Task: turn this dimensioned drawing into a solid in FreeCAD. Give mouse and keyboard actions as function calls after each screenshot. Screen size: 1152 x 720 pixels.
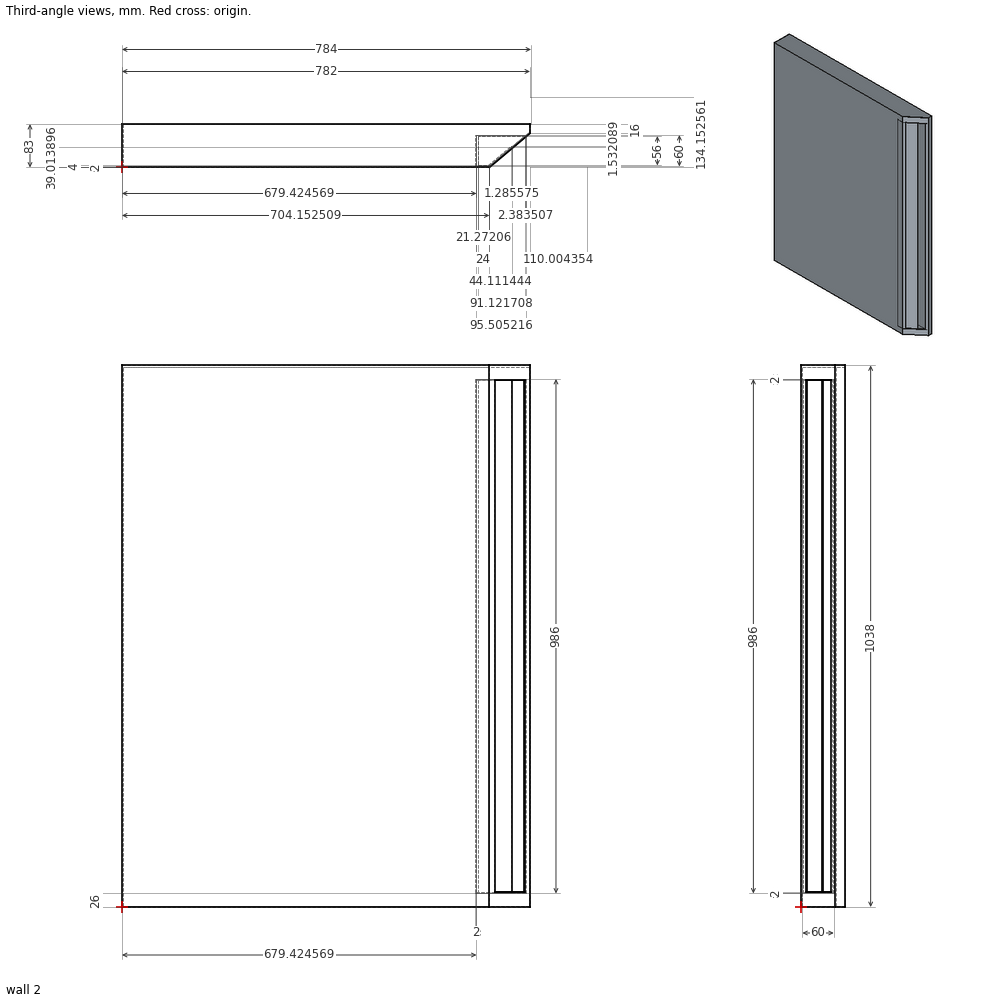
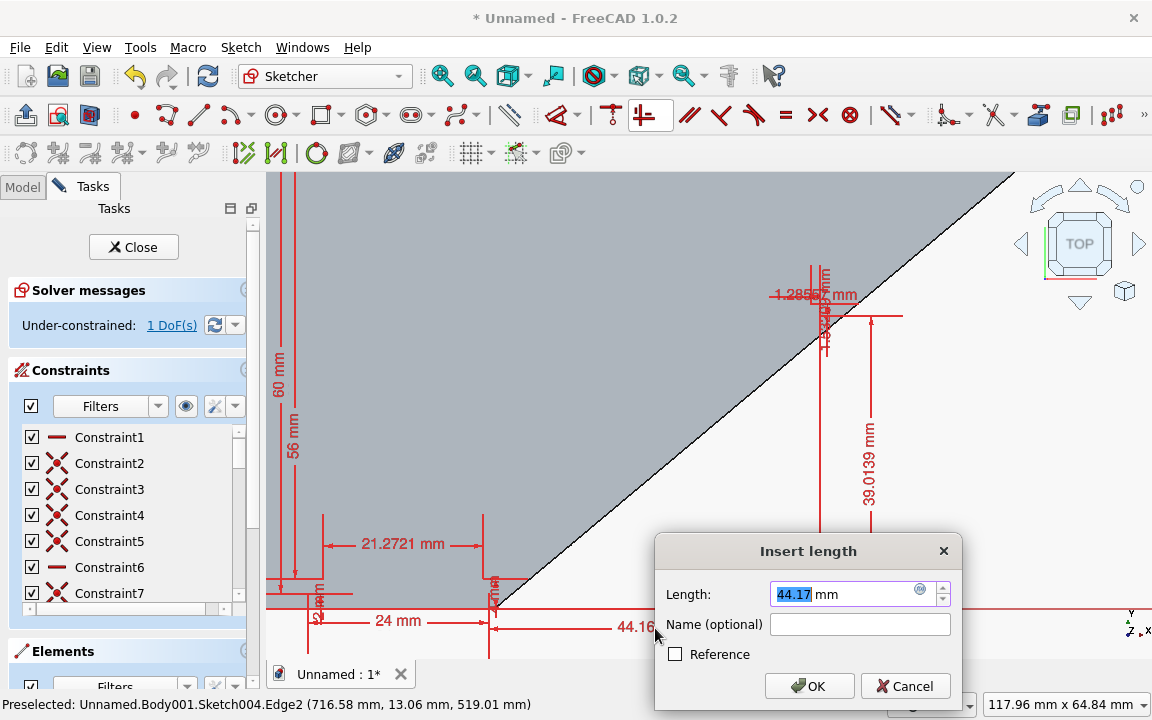
text(44.111444)
key(Return)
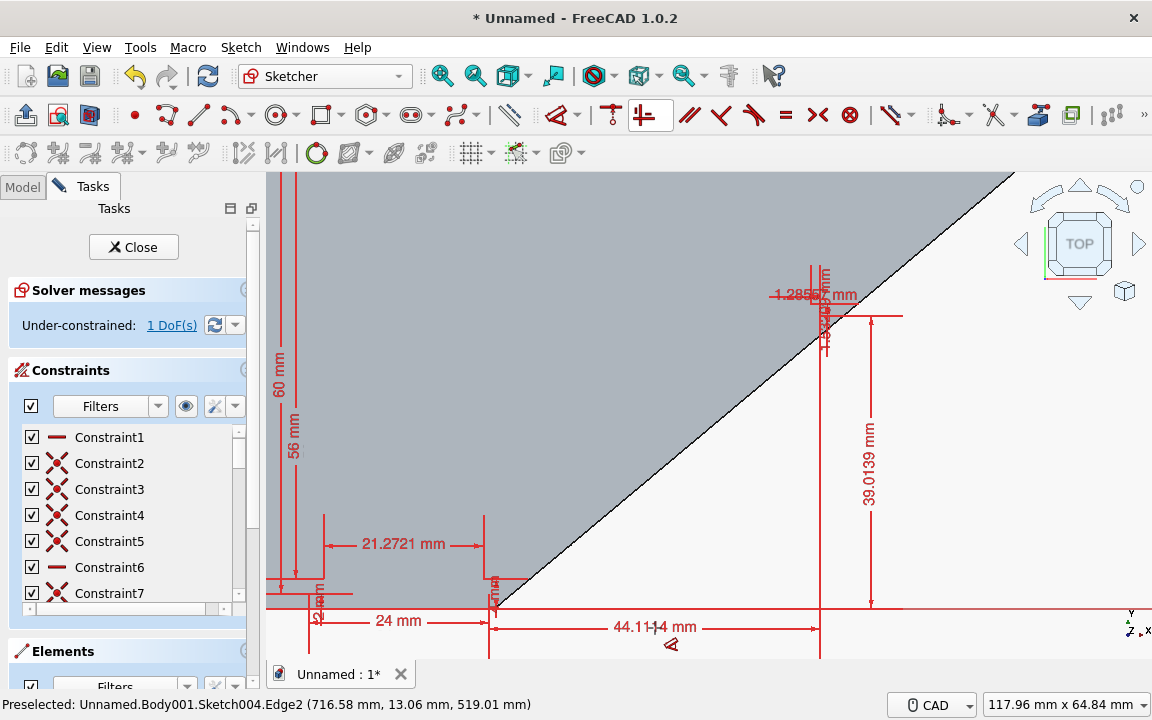
click(309, 594)
click(301, 560)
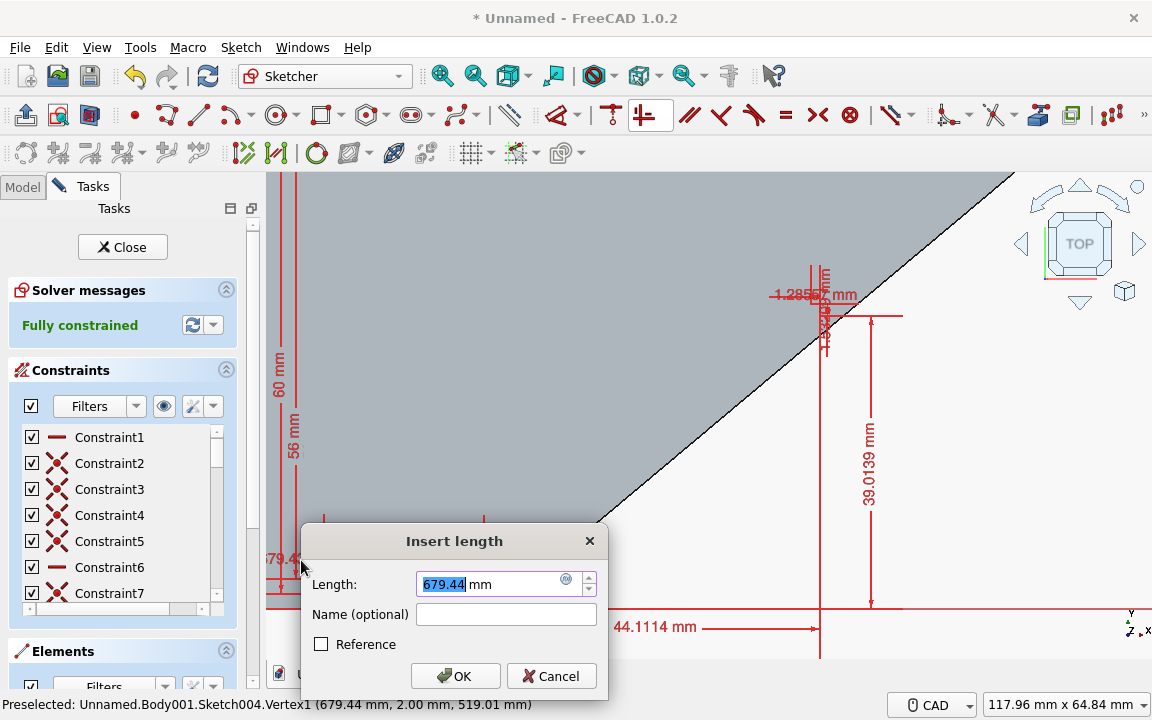
text(679.424569)
key(Return)
key(Escape)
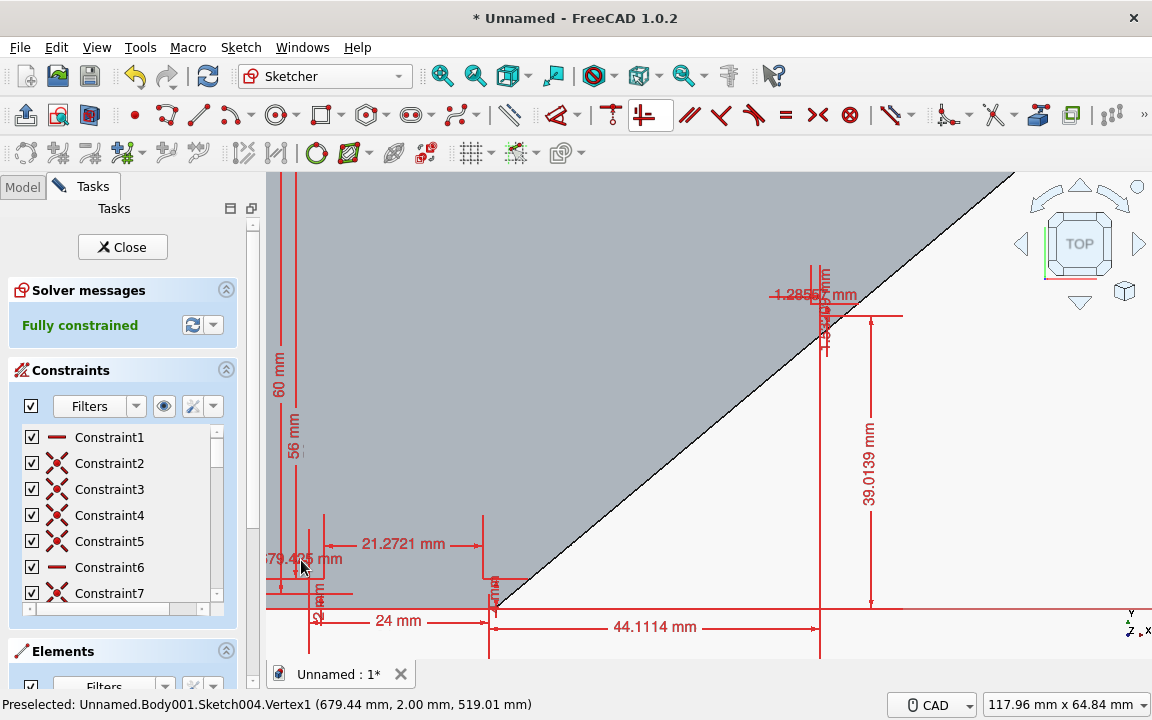
click(123, 247)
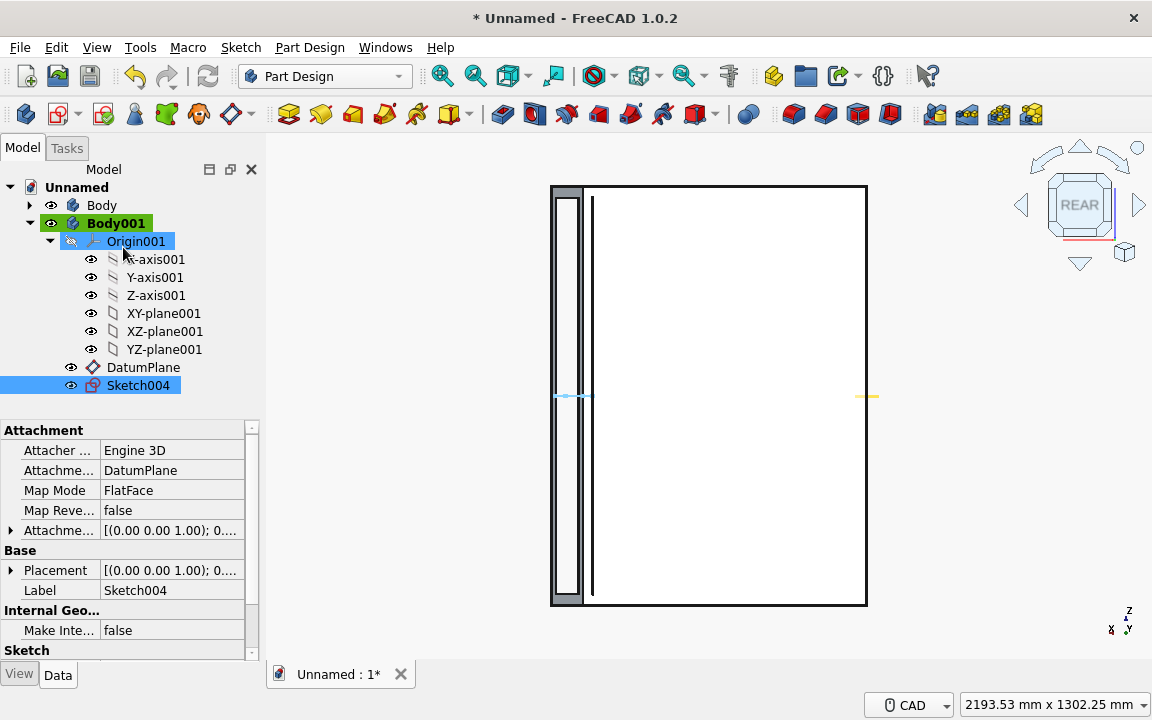
click(290, 114)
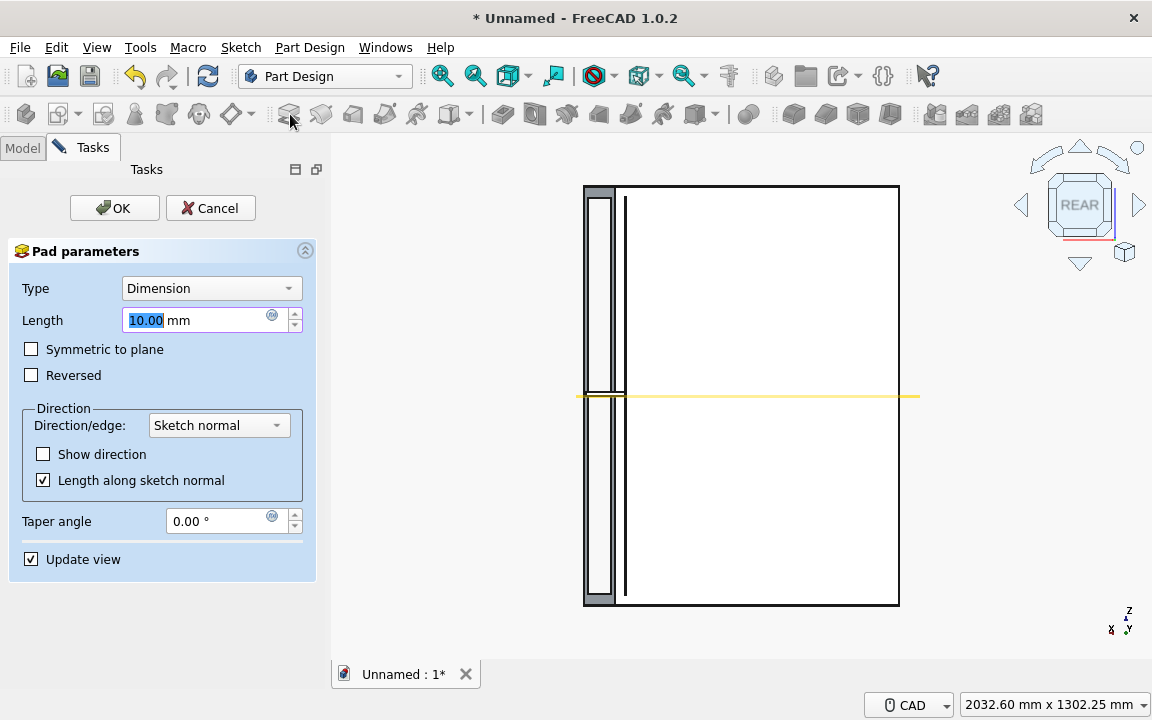
text(986)
key(Tab)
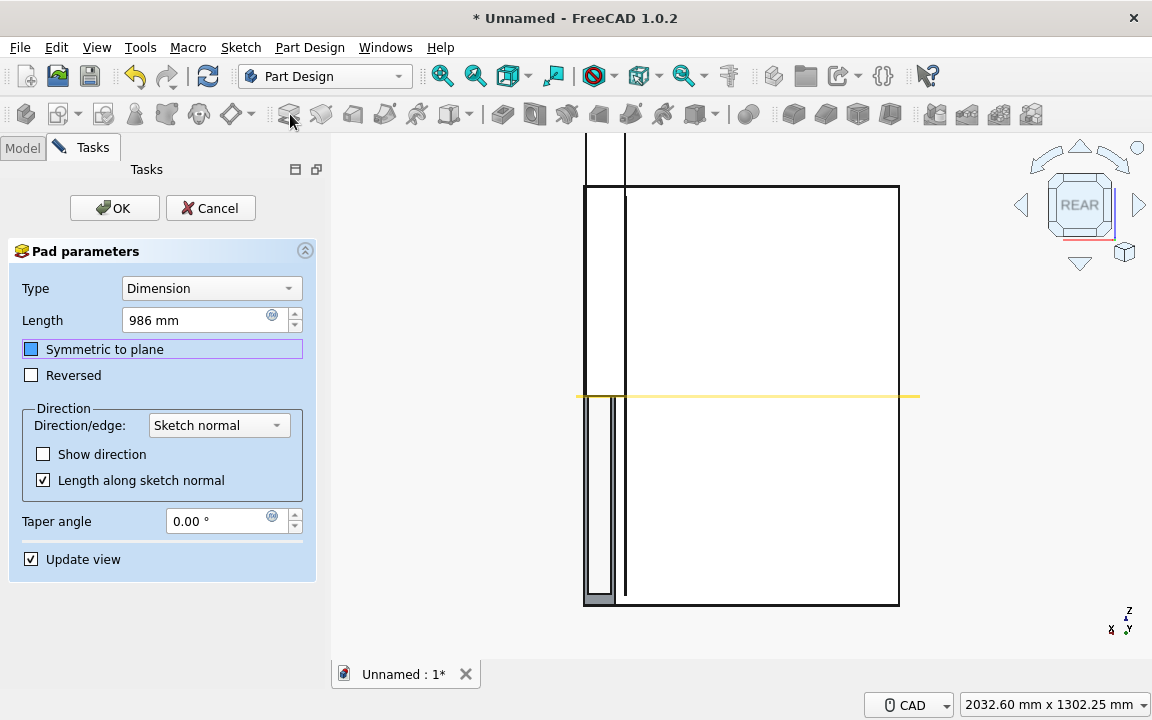
click(30, 349)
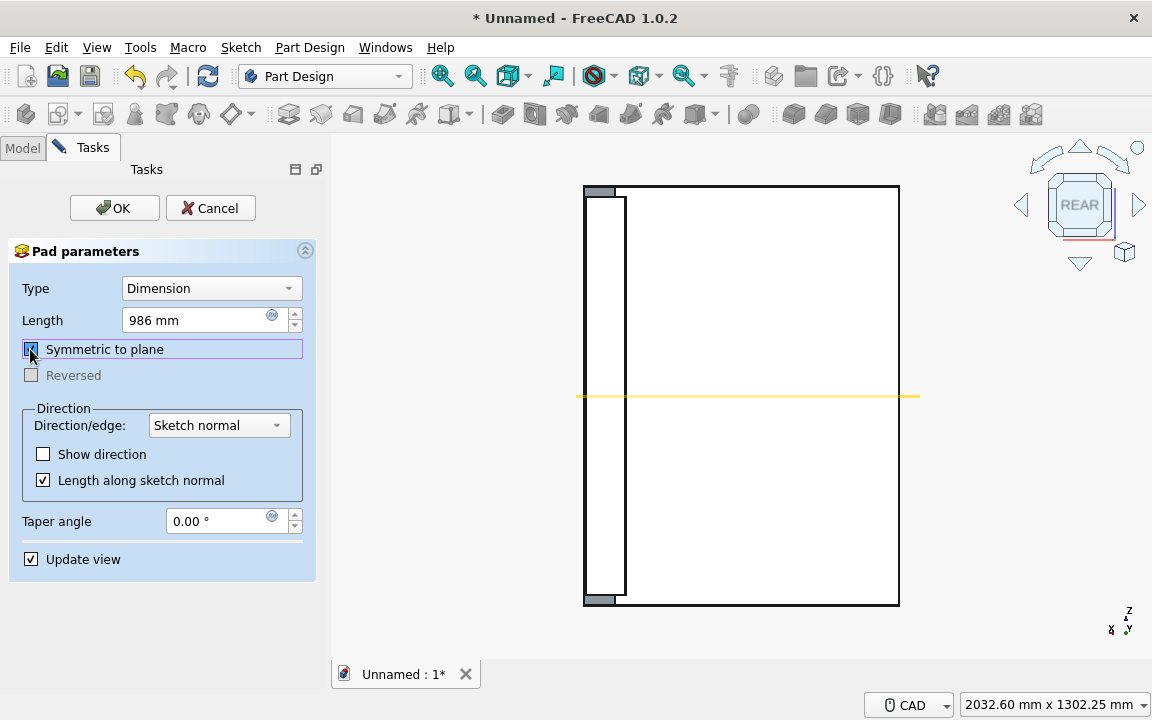
click(115, 208)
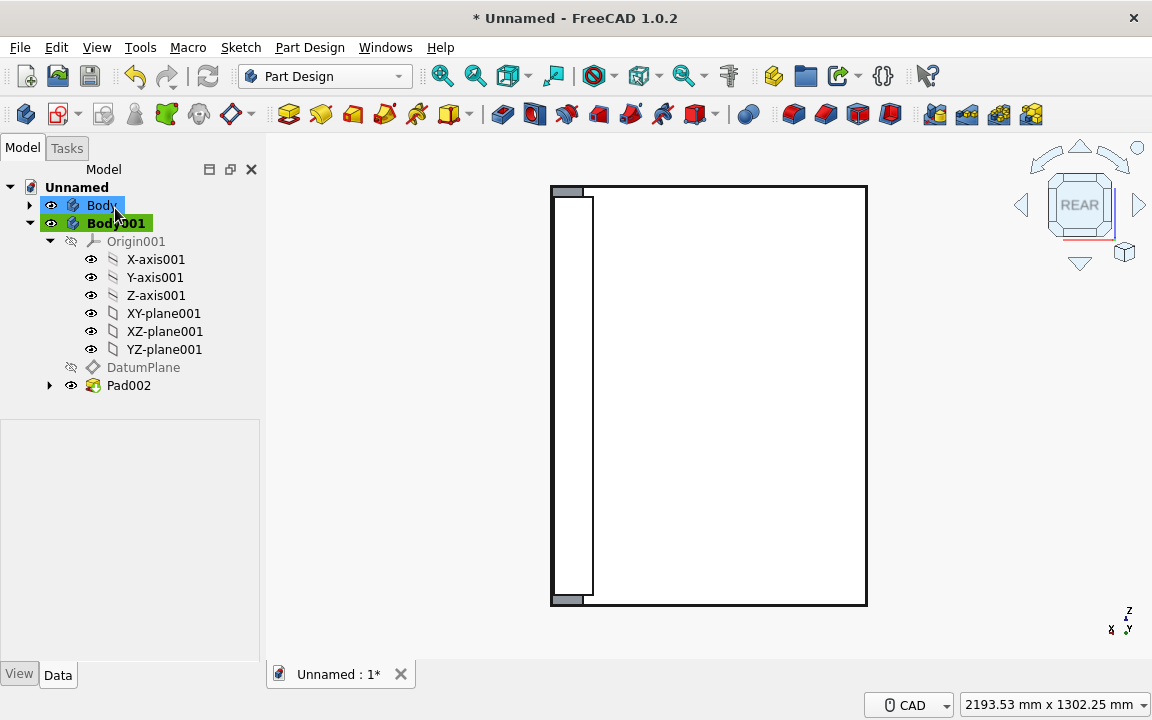
click(26, 114)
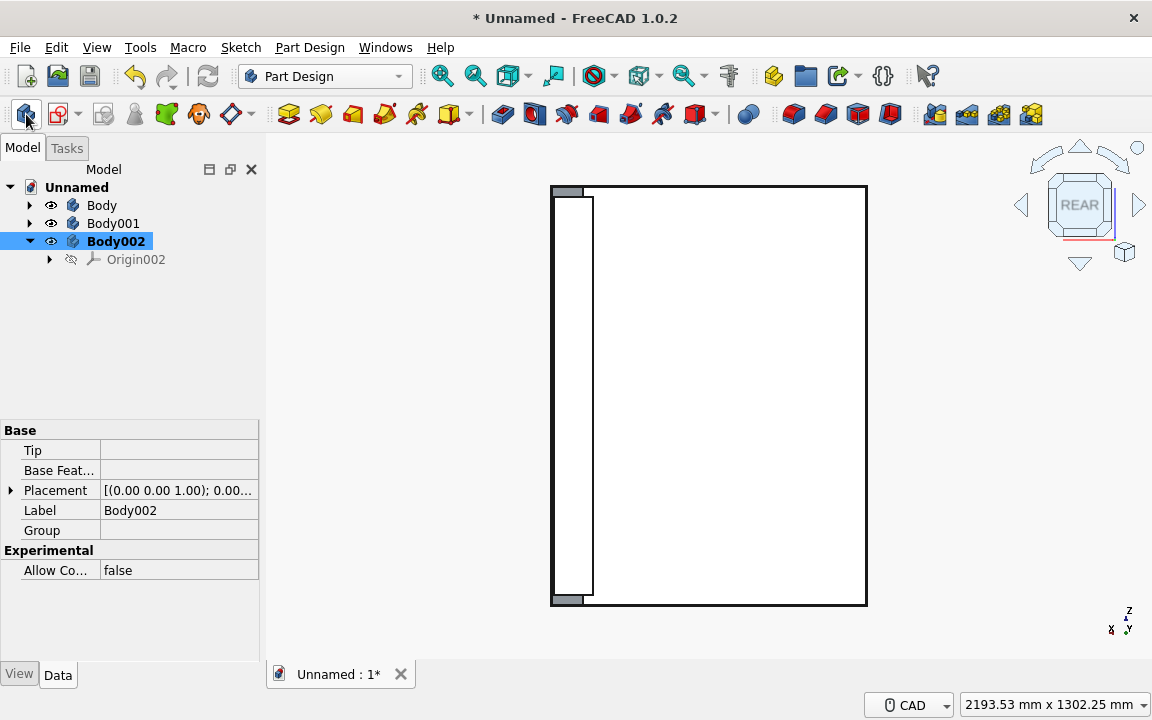
click(50, 259)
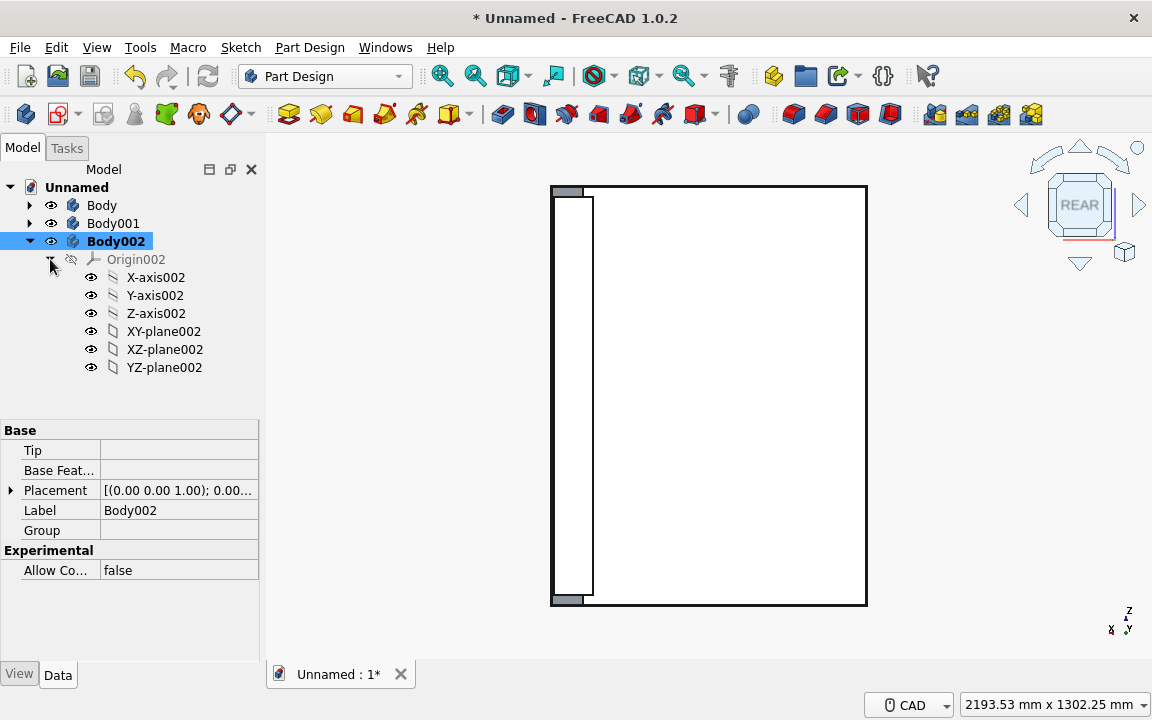
click(136, 331)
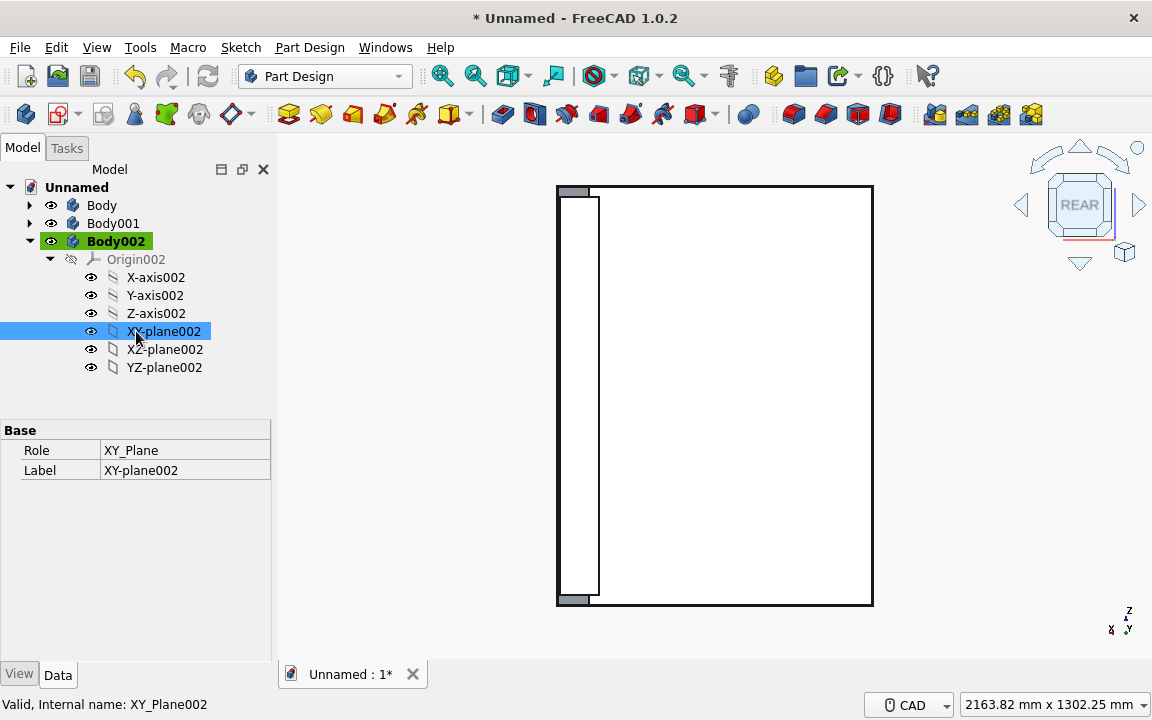
click(232, 114)